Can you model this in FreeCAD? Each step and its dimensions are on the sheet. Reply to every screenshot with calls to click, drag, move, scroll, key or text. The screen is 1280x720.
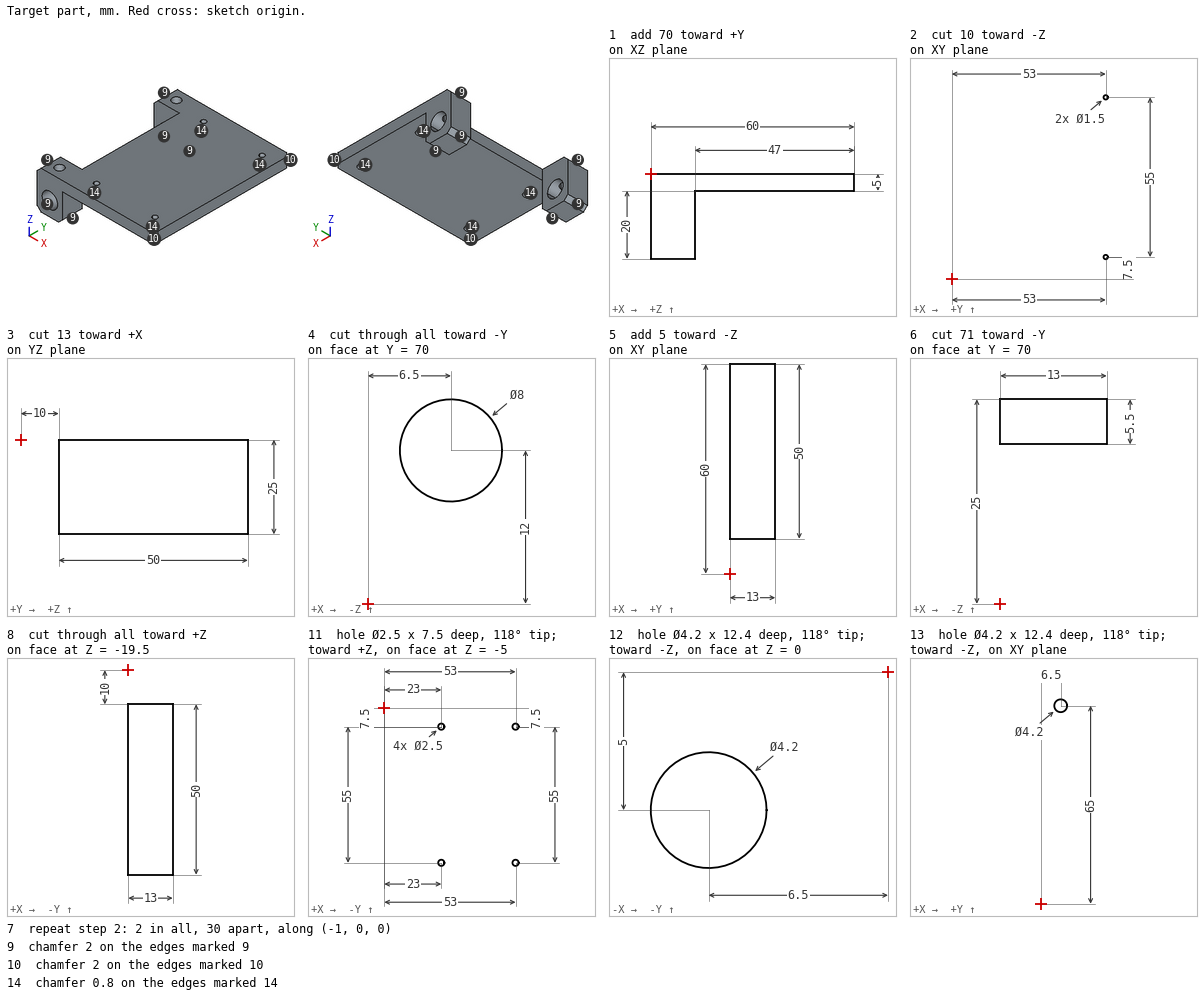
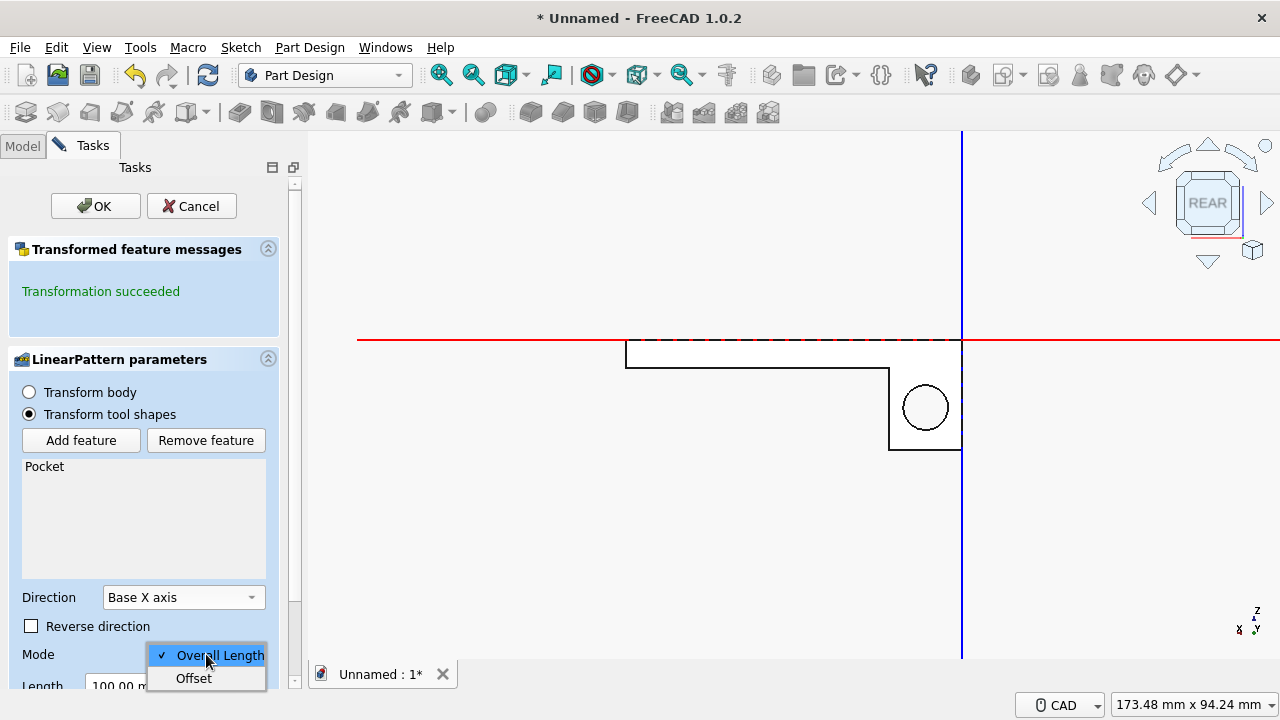
click(206, 678)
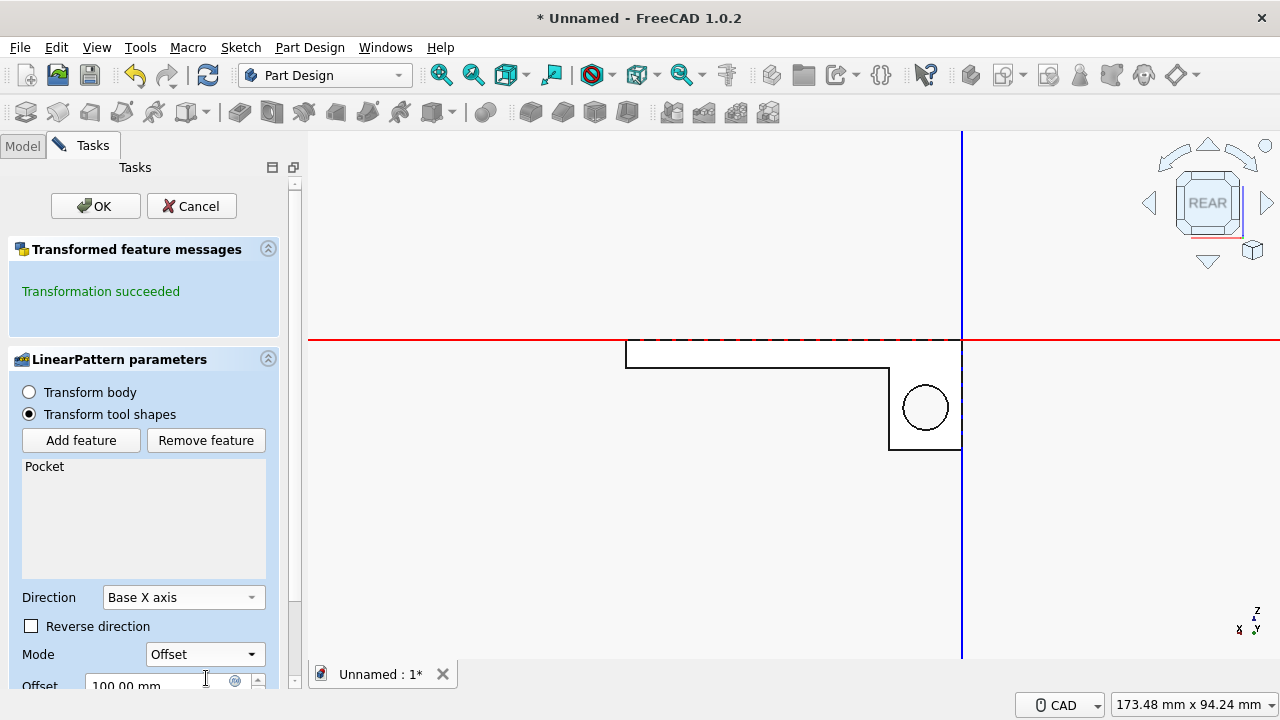
scroll(295, 432, down, 2)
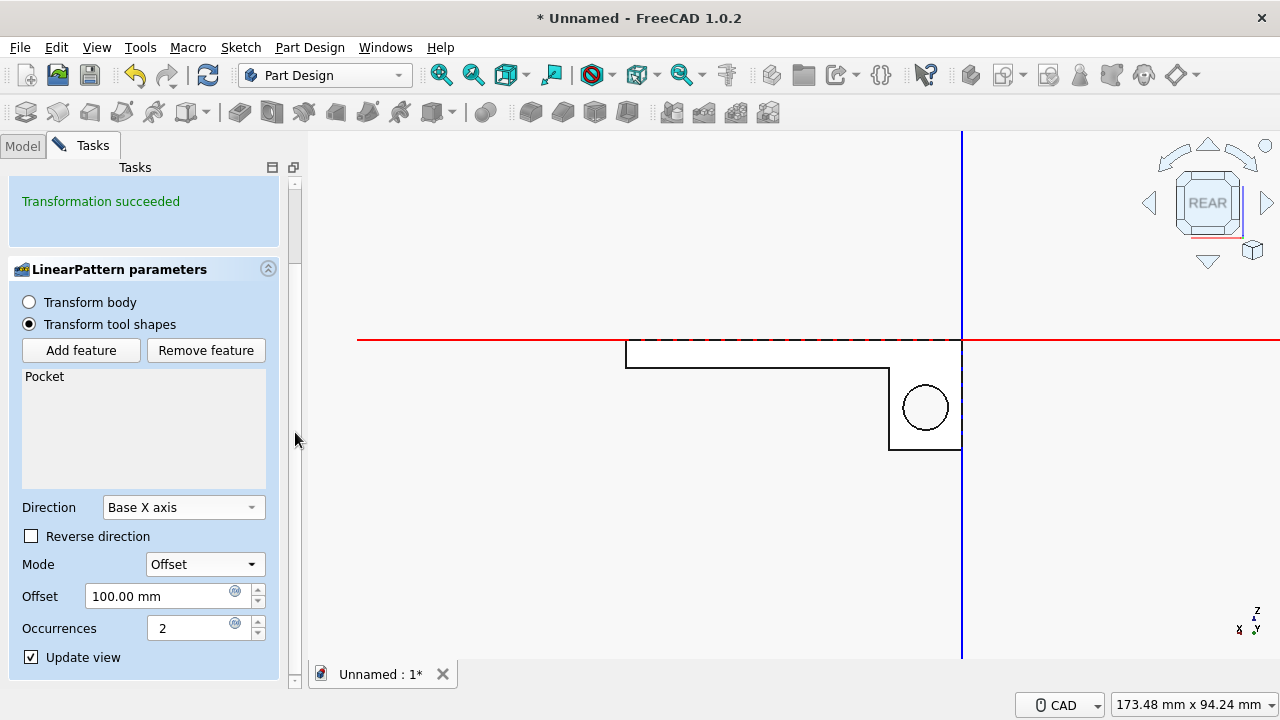
triple_click(168, 596)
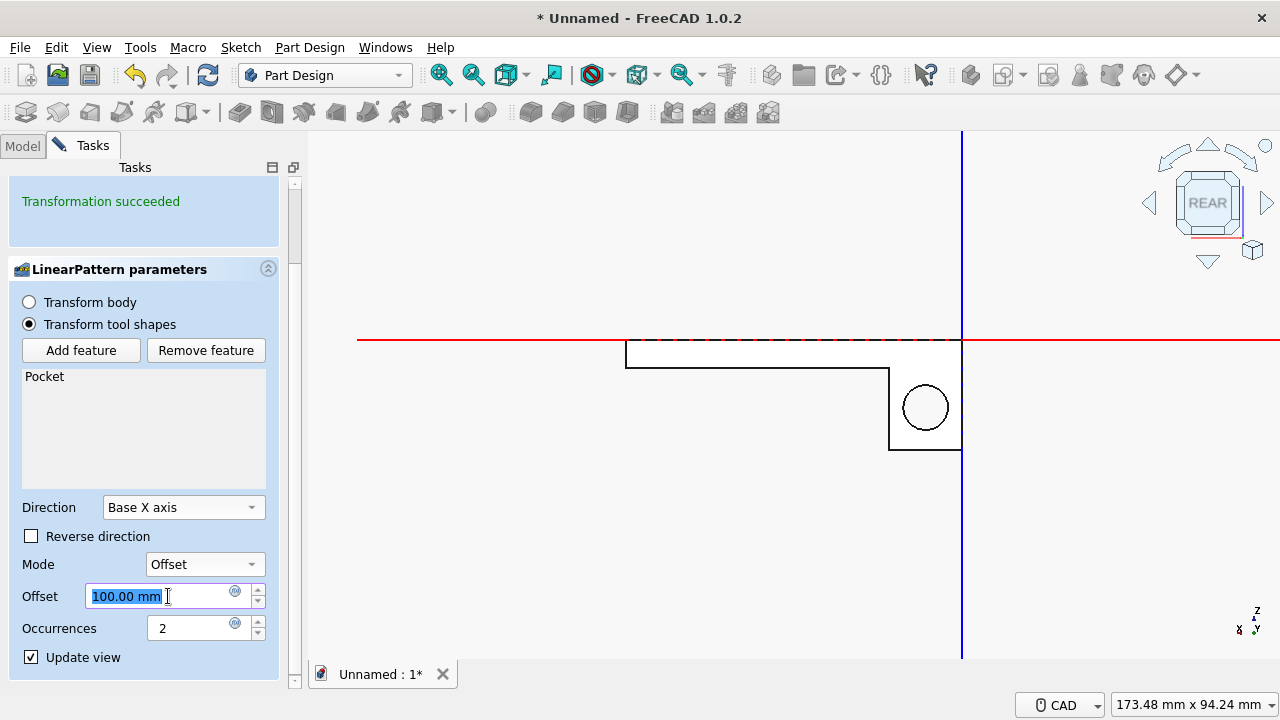
text(30)
key(Tab)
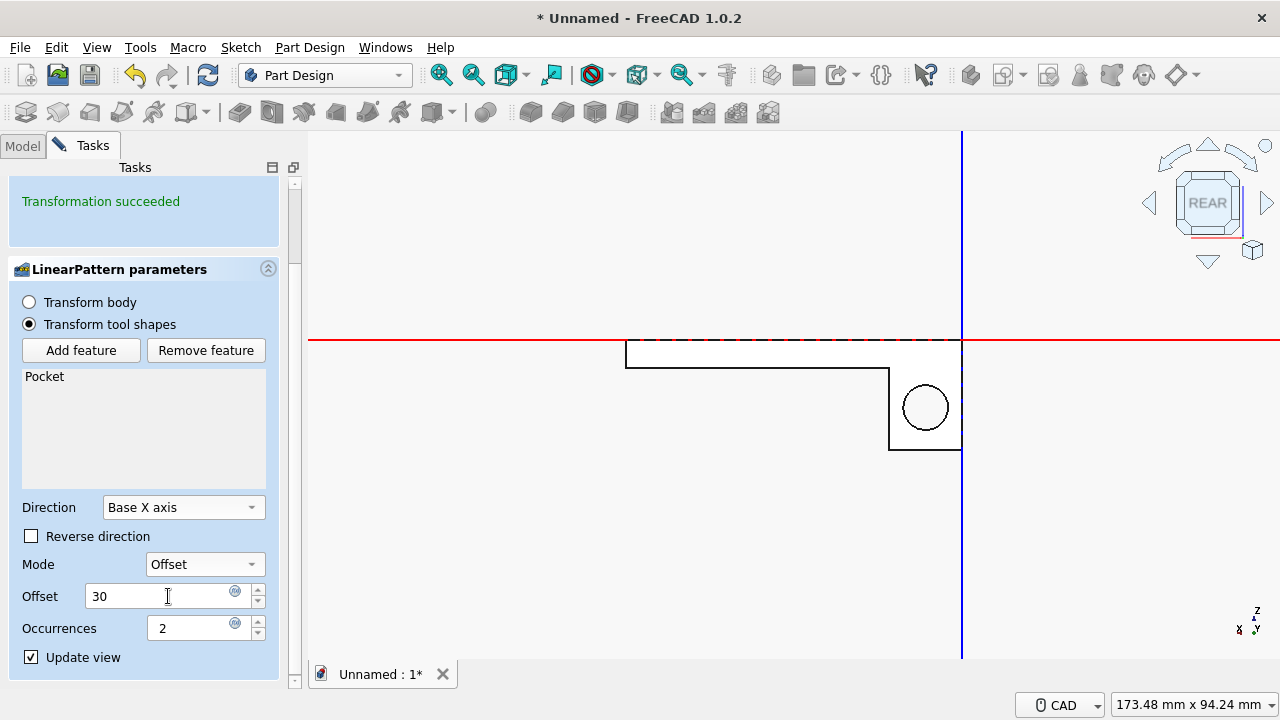
triple_click(198, 628)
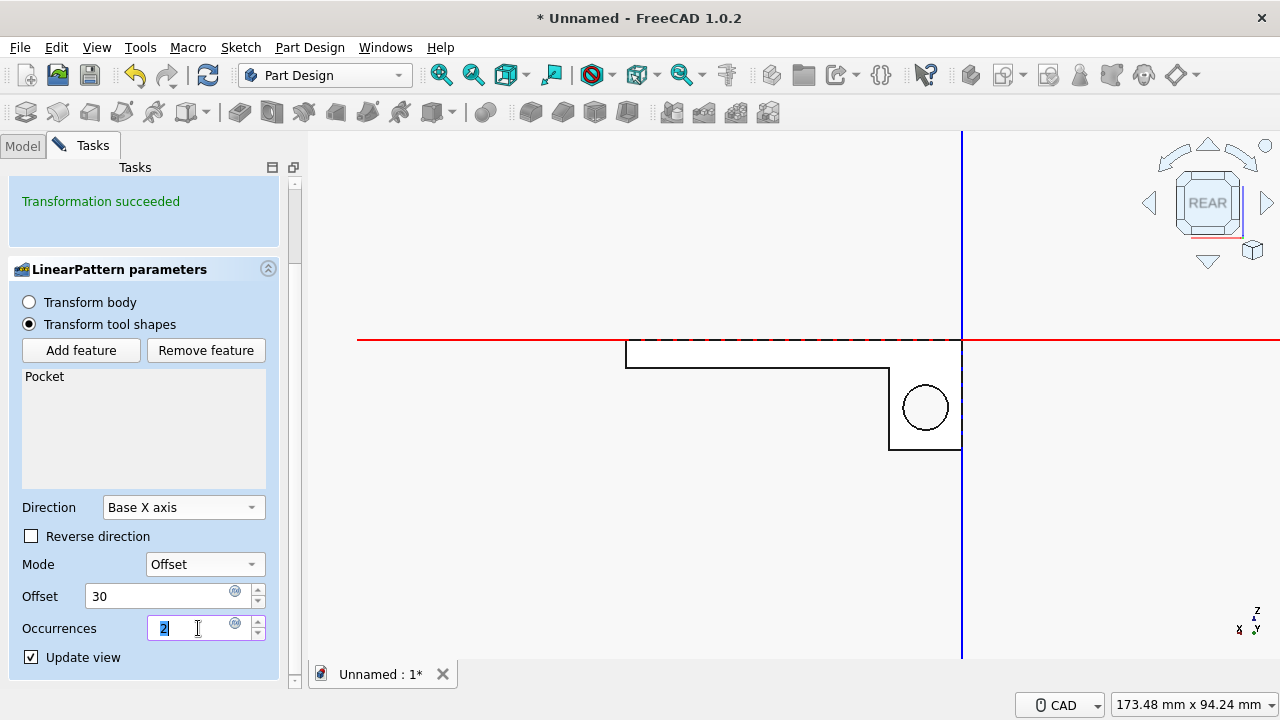
text(2)
key(Tab)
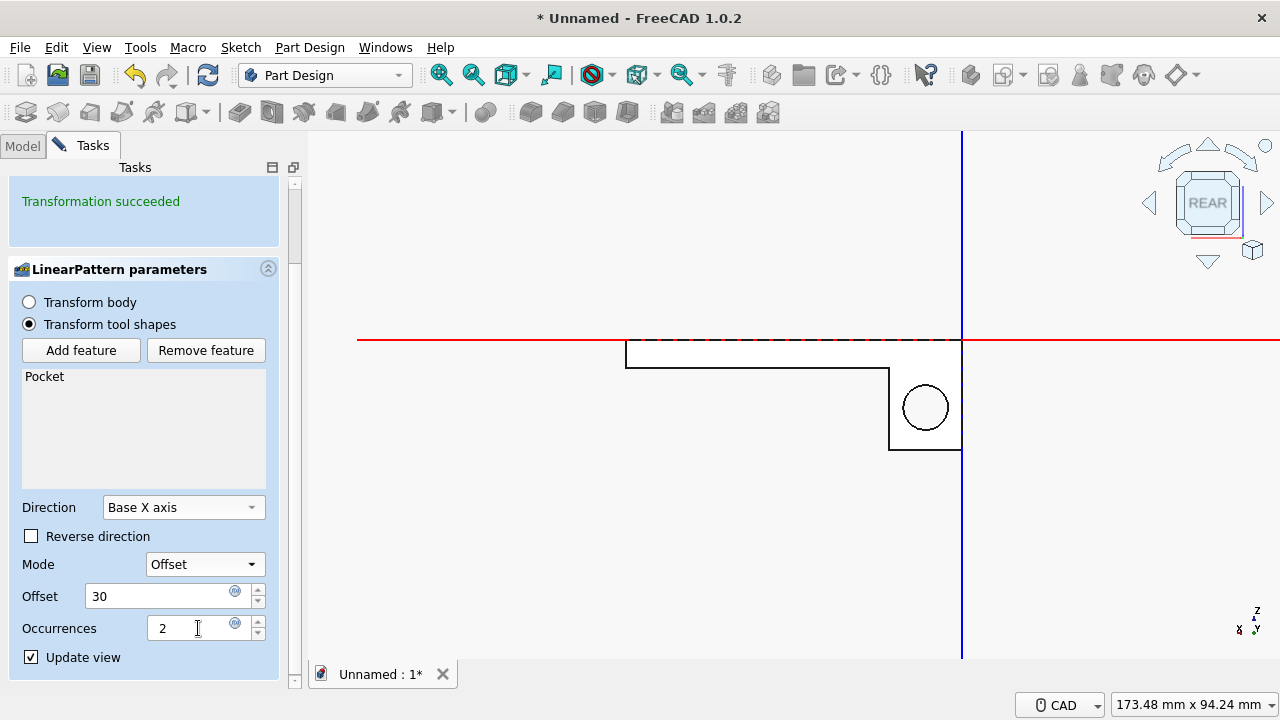
click(30, 536)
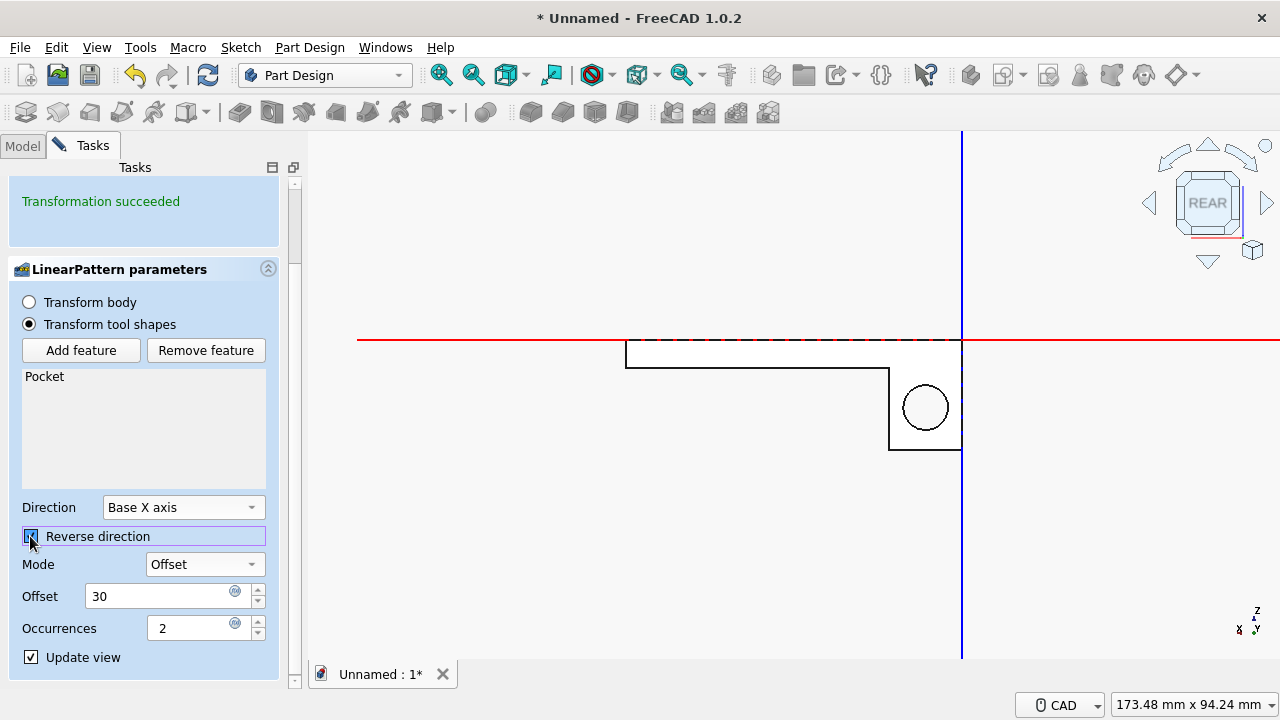
scroll(295, 432, up, 3)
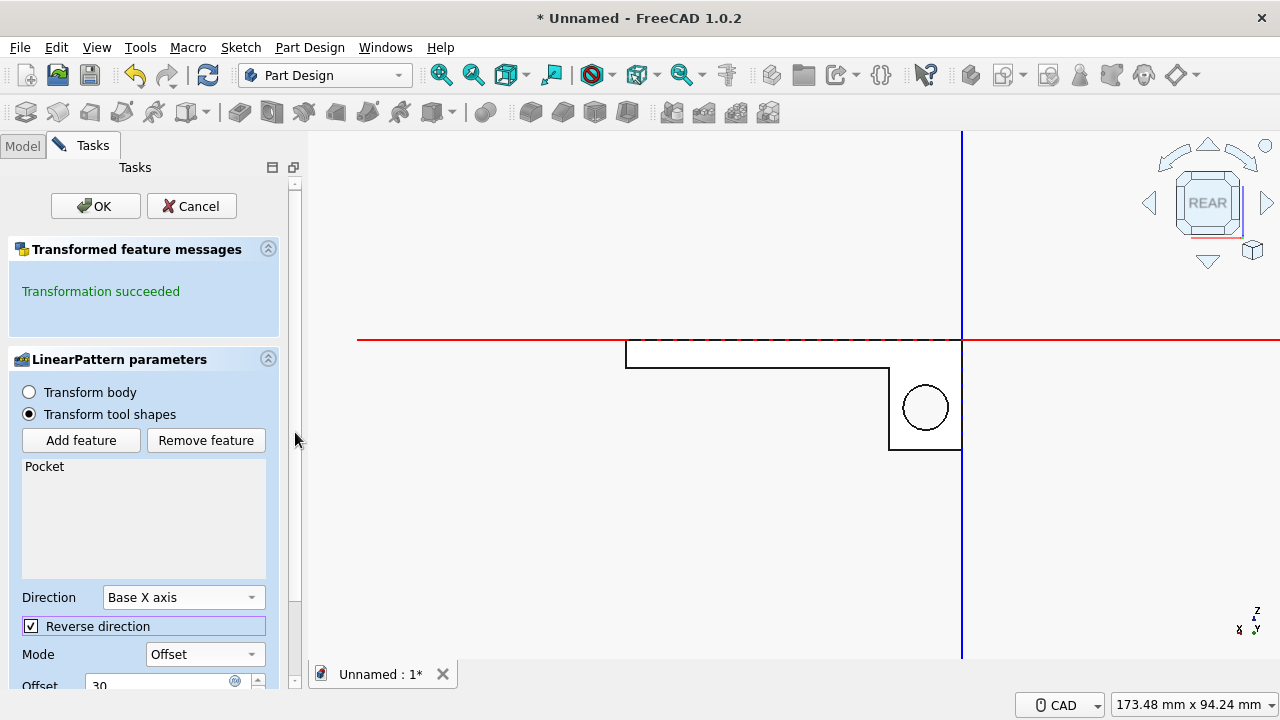
click(96, 206)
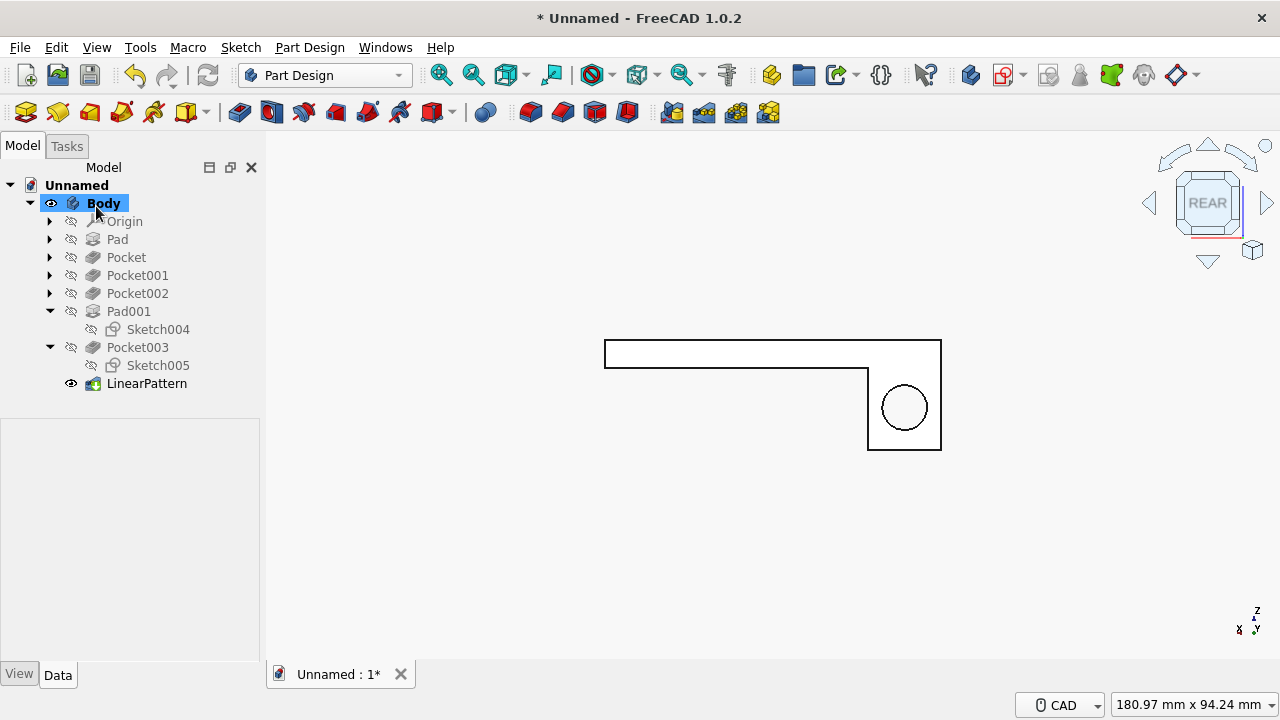
click(442, 76)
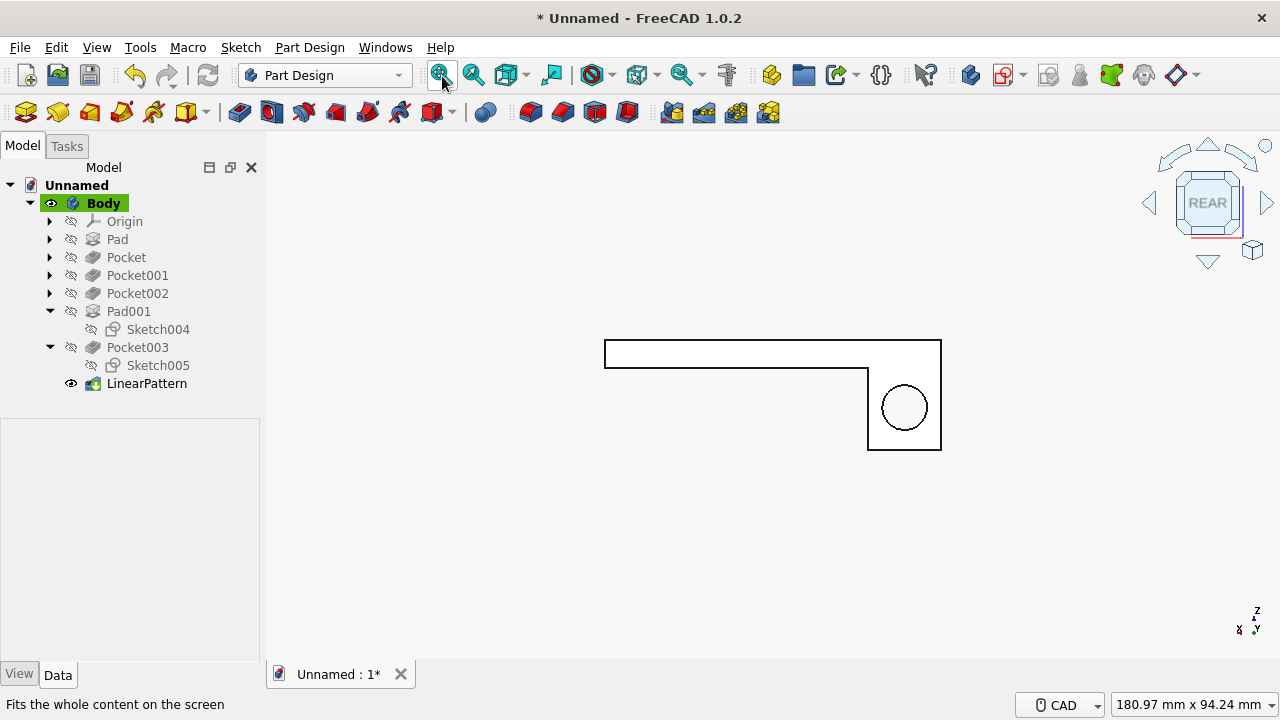
key(5)